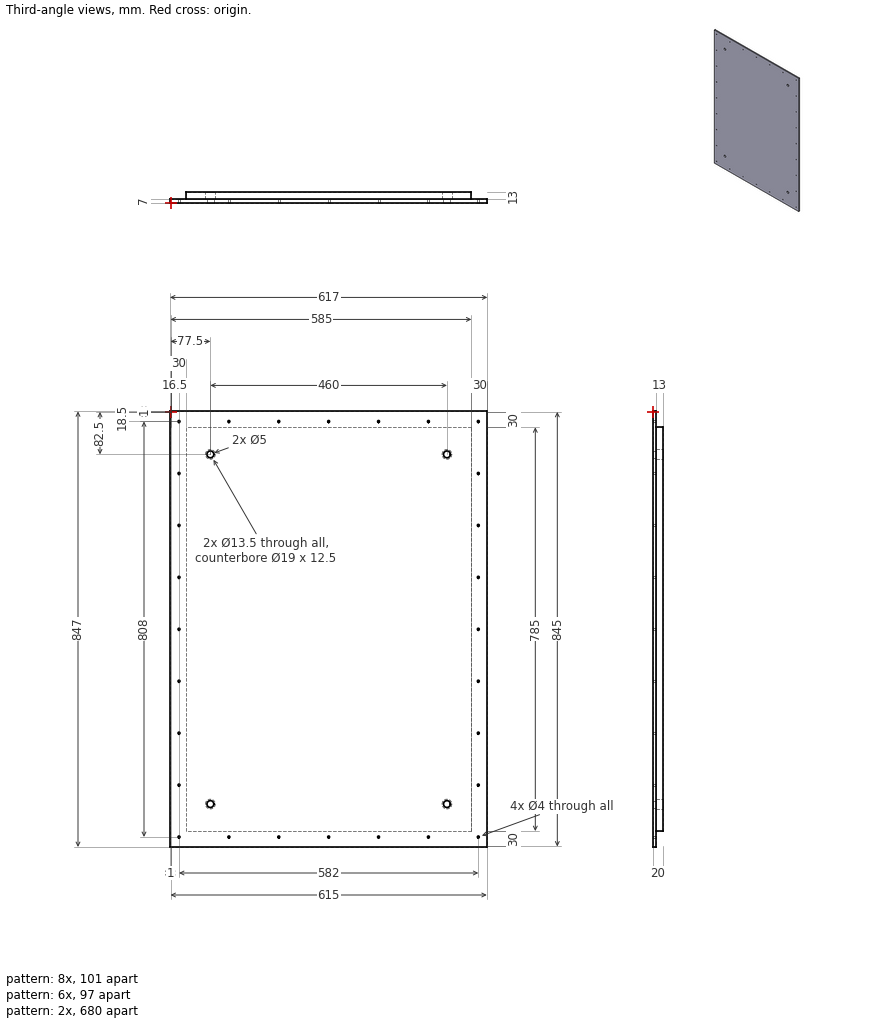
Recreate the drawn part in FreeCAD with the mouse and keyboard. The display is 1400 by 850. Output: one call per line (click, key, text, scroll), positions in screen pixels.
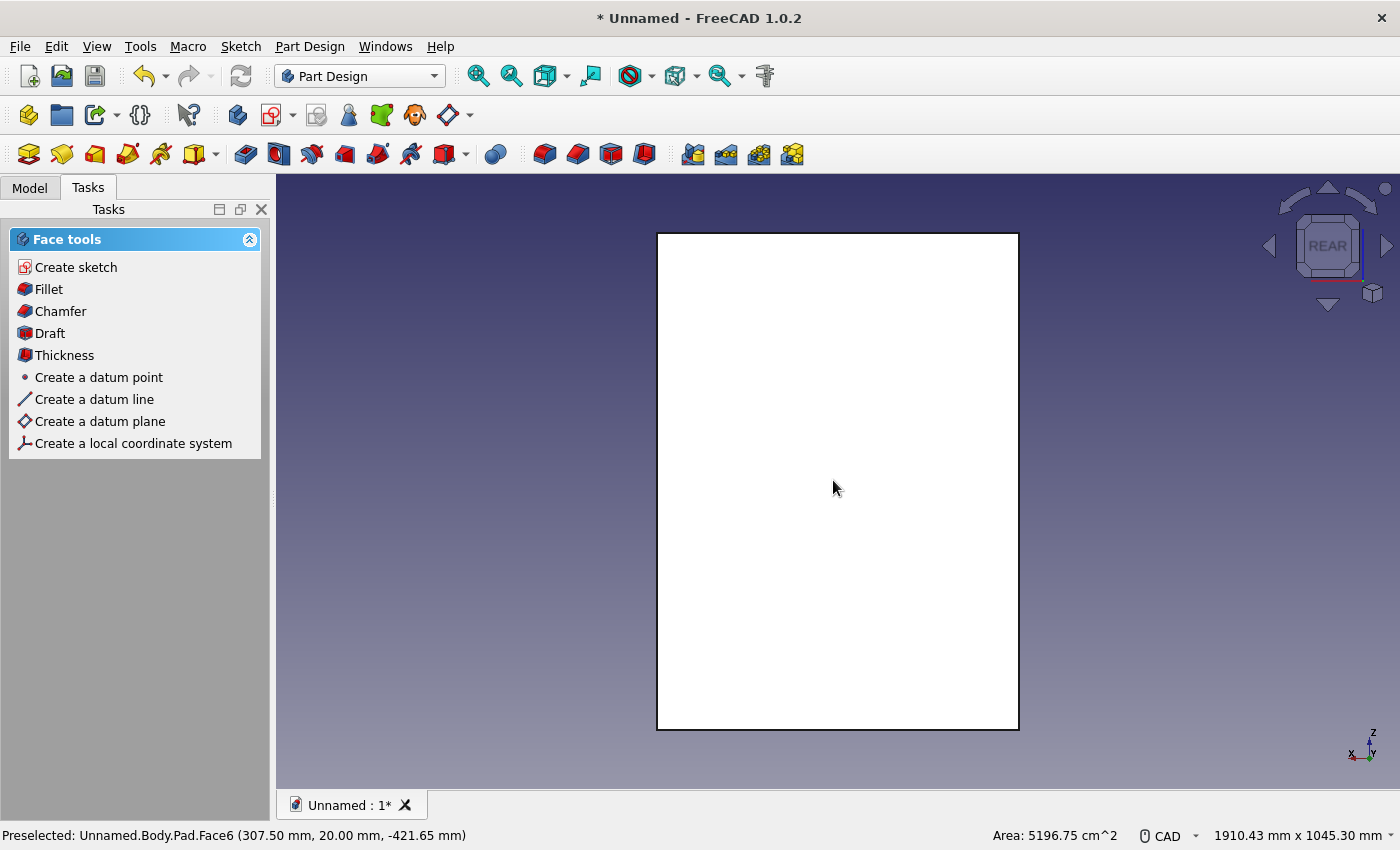
click(270, 116)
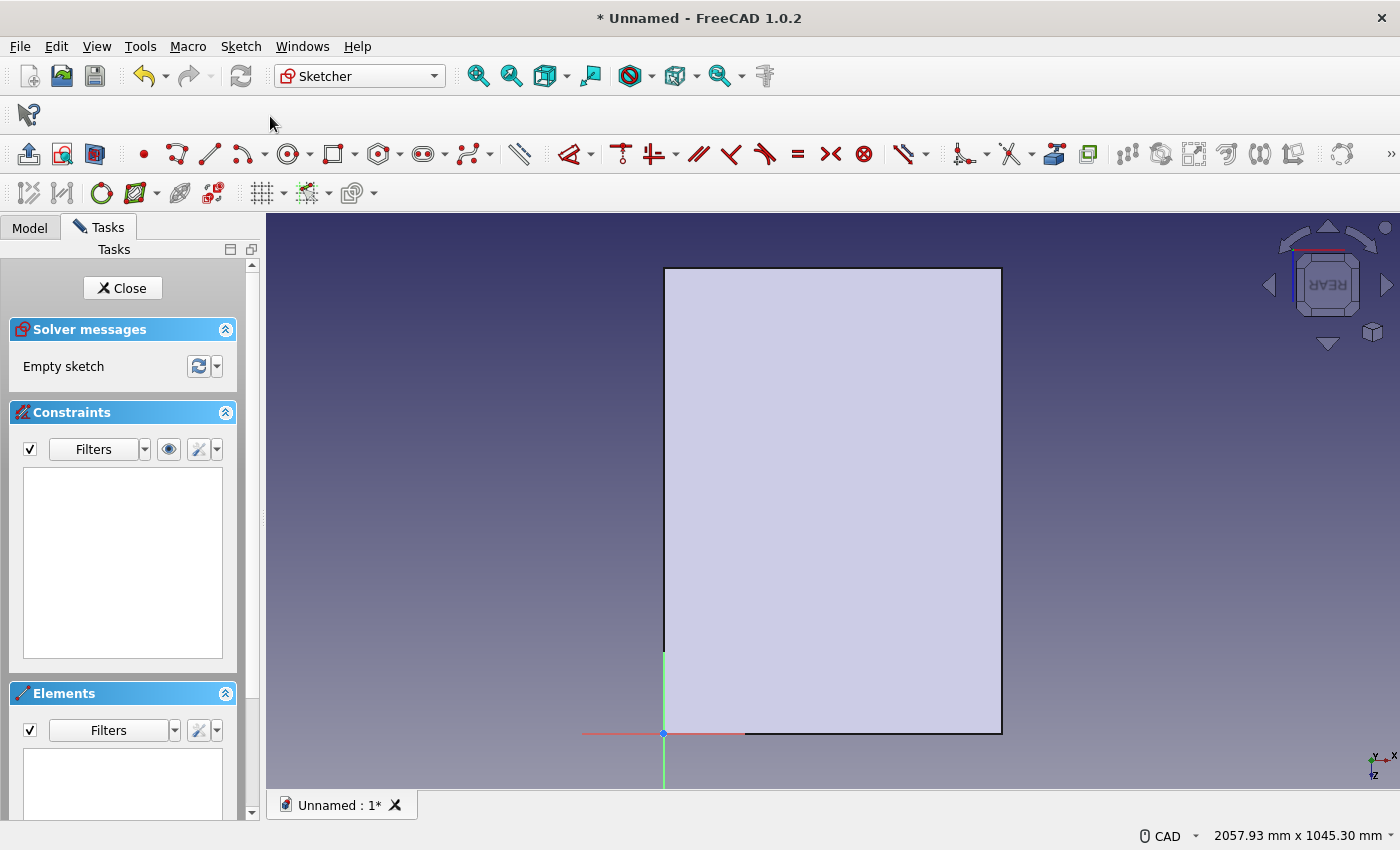
click(332, 154)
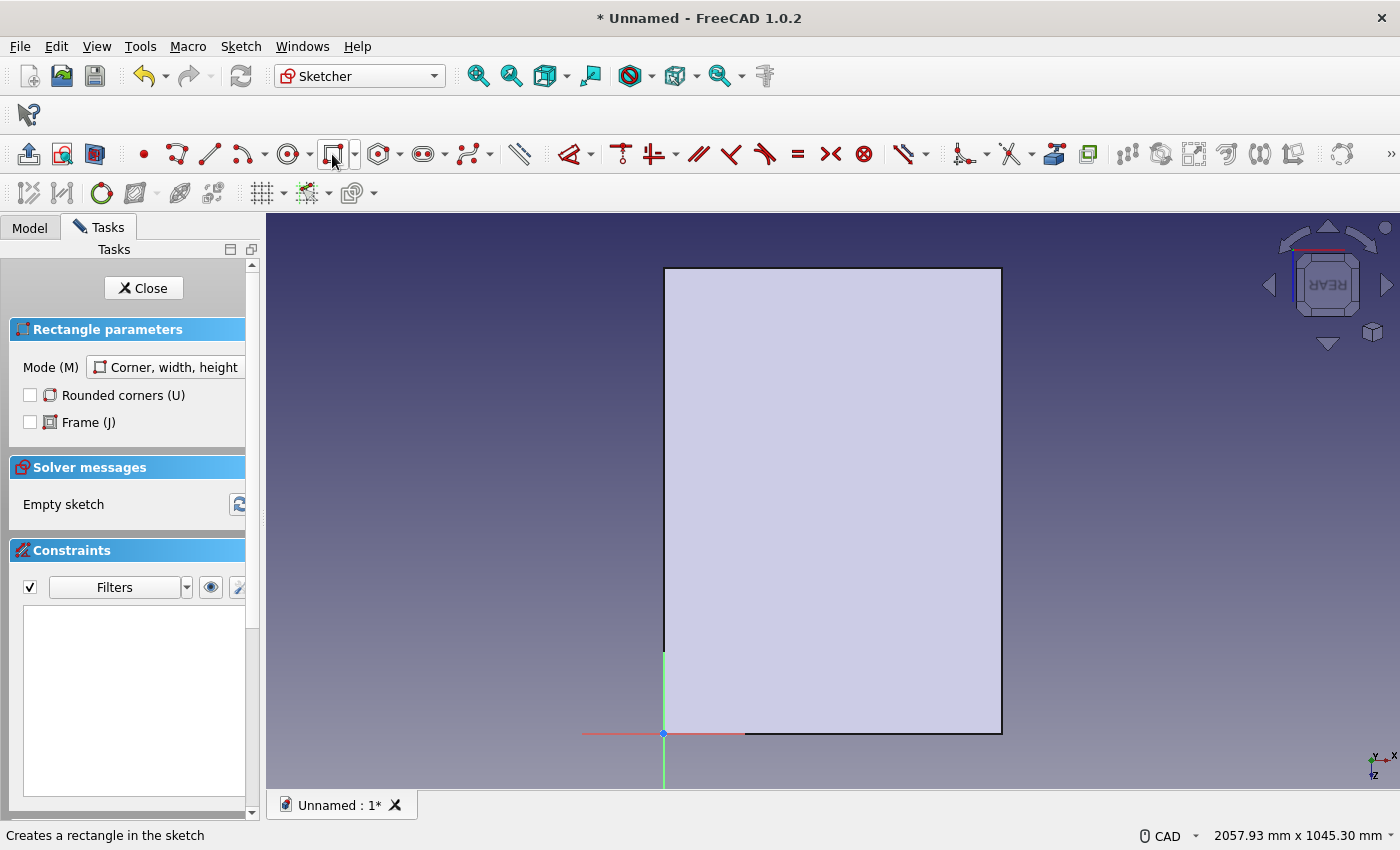
click(664, 268)
move(1002, 285)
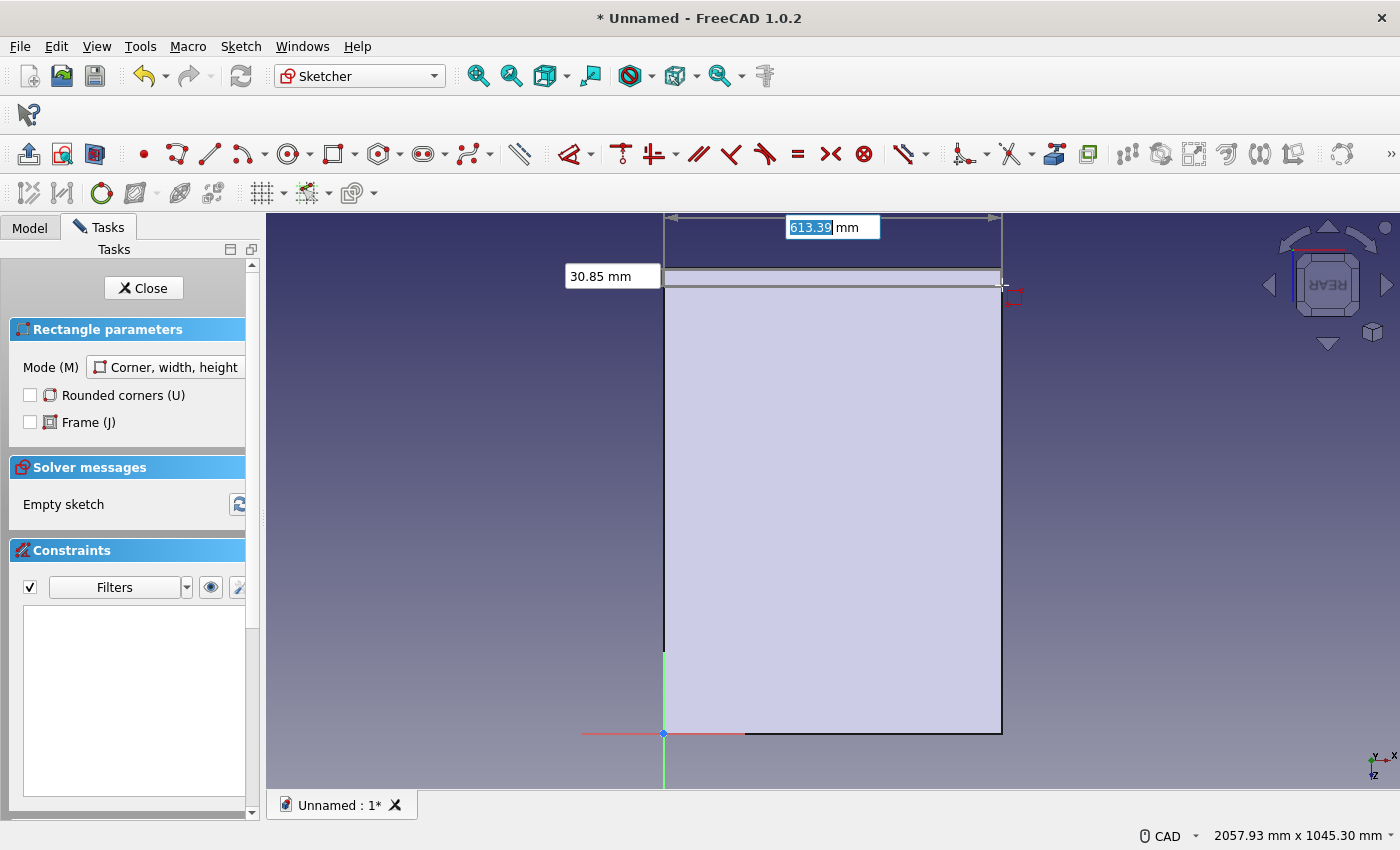
text(615)
key(Tab)
text(30)
key(Return)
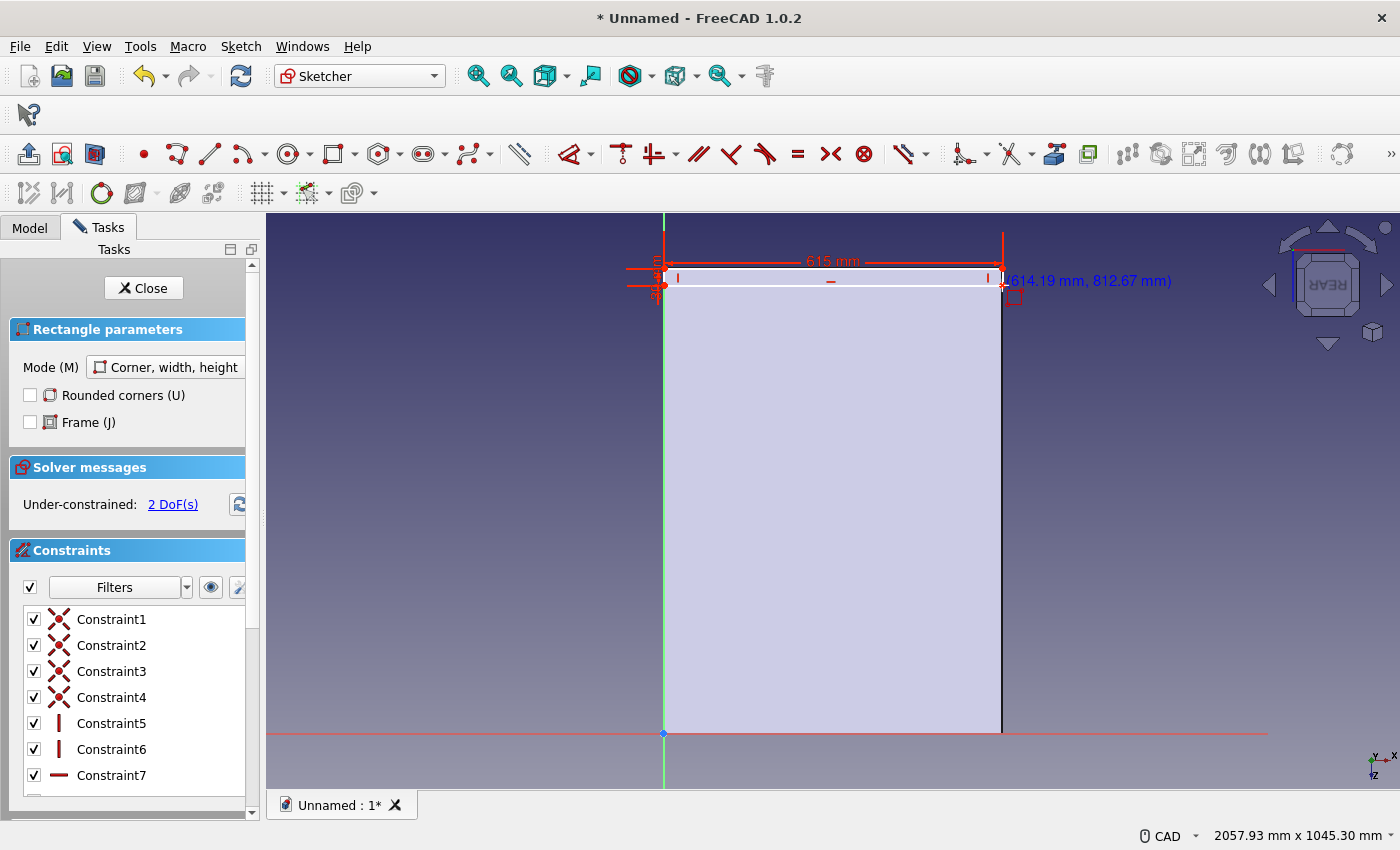
click(664, 734)
move(1002, 717)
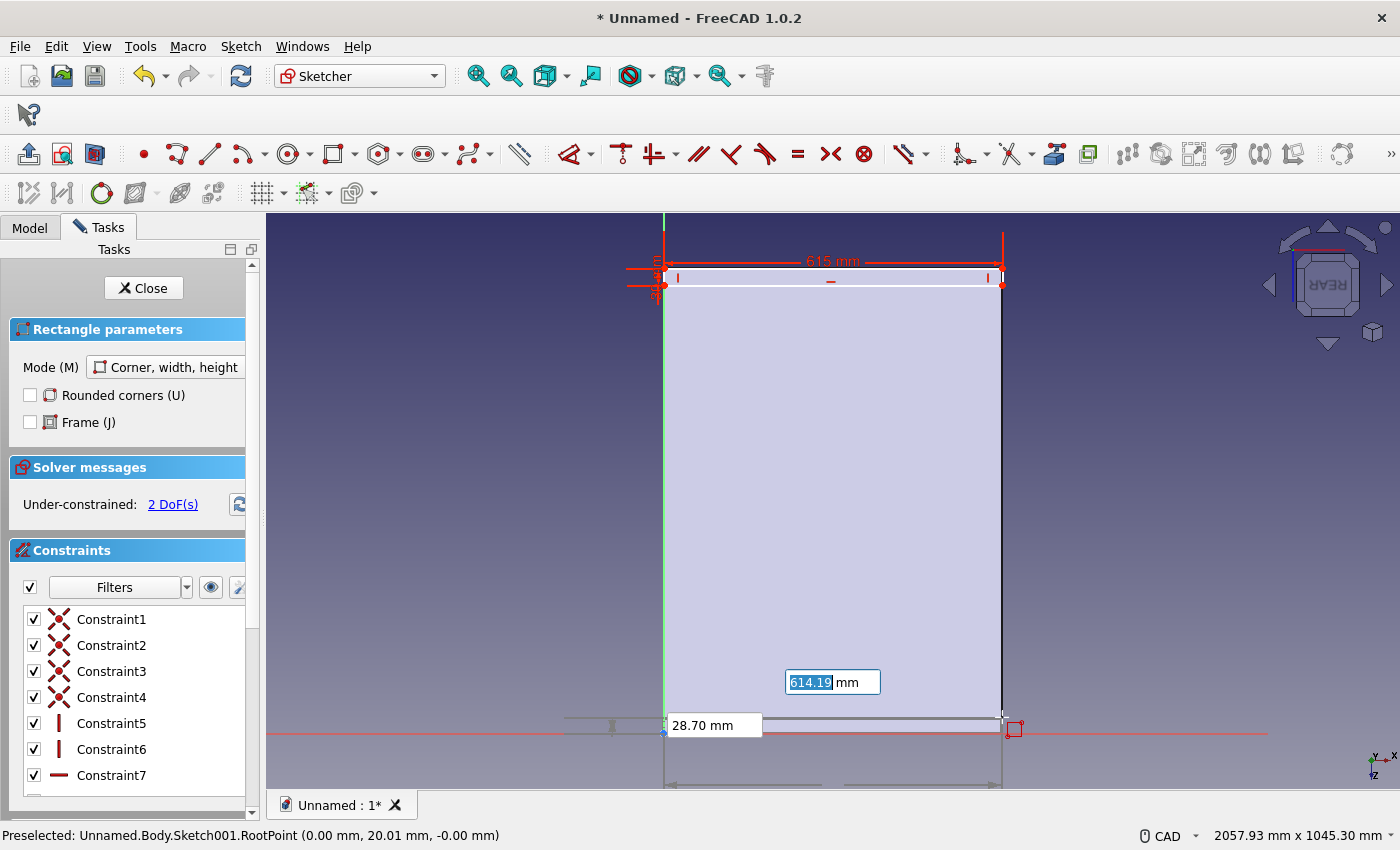
text(615)
key(Tab)
text(30)
key(Return)
key(Escape)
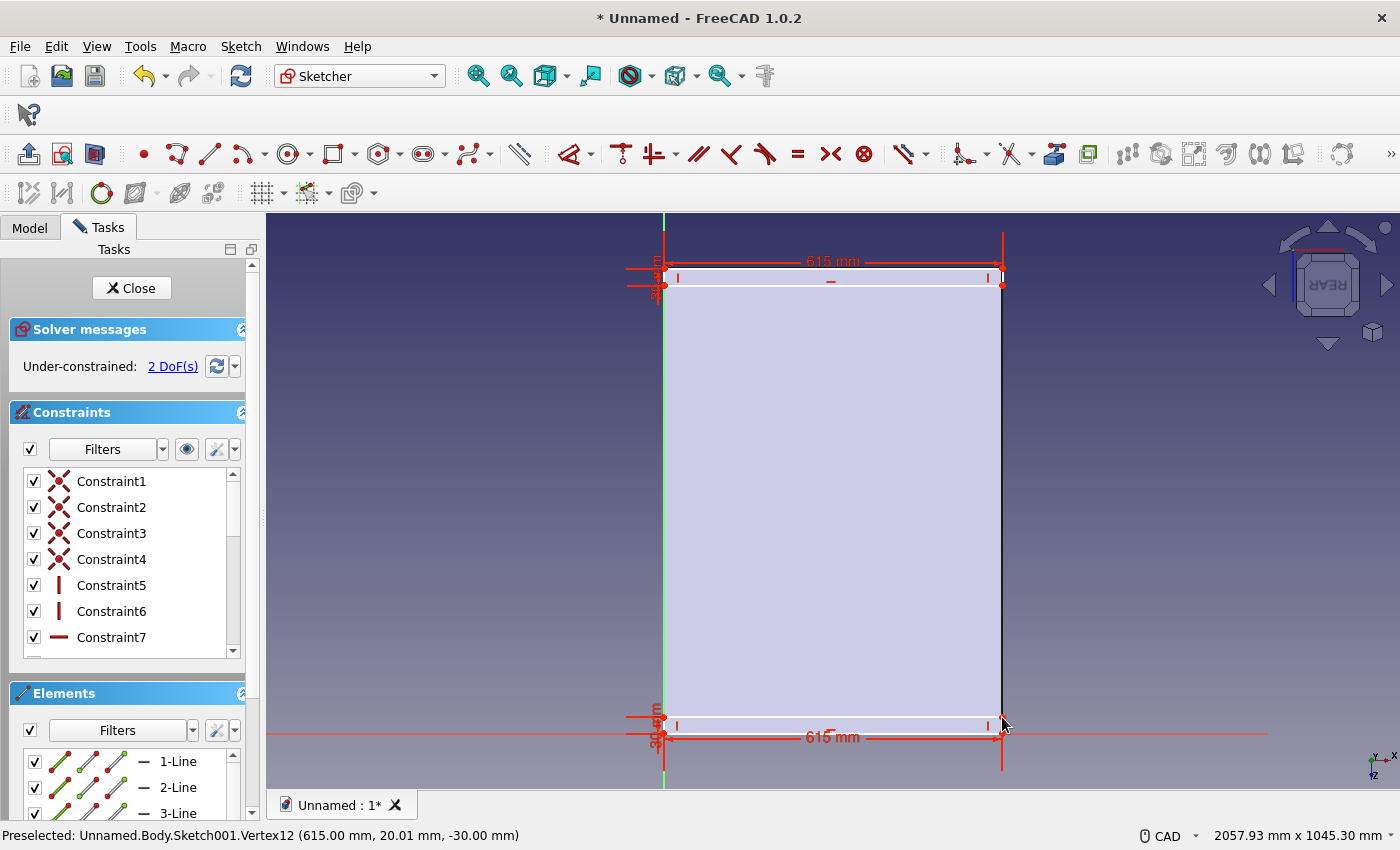
click(664, 269)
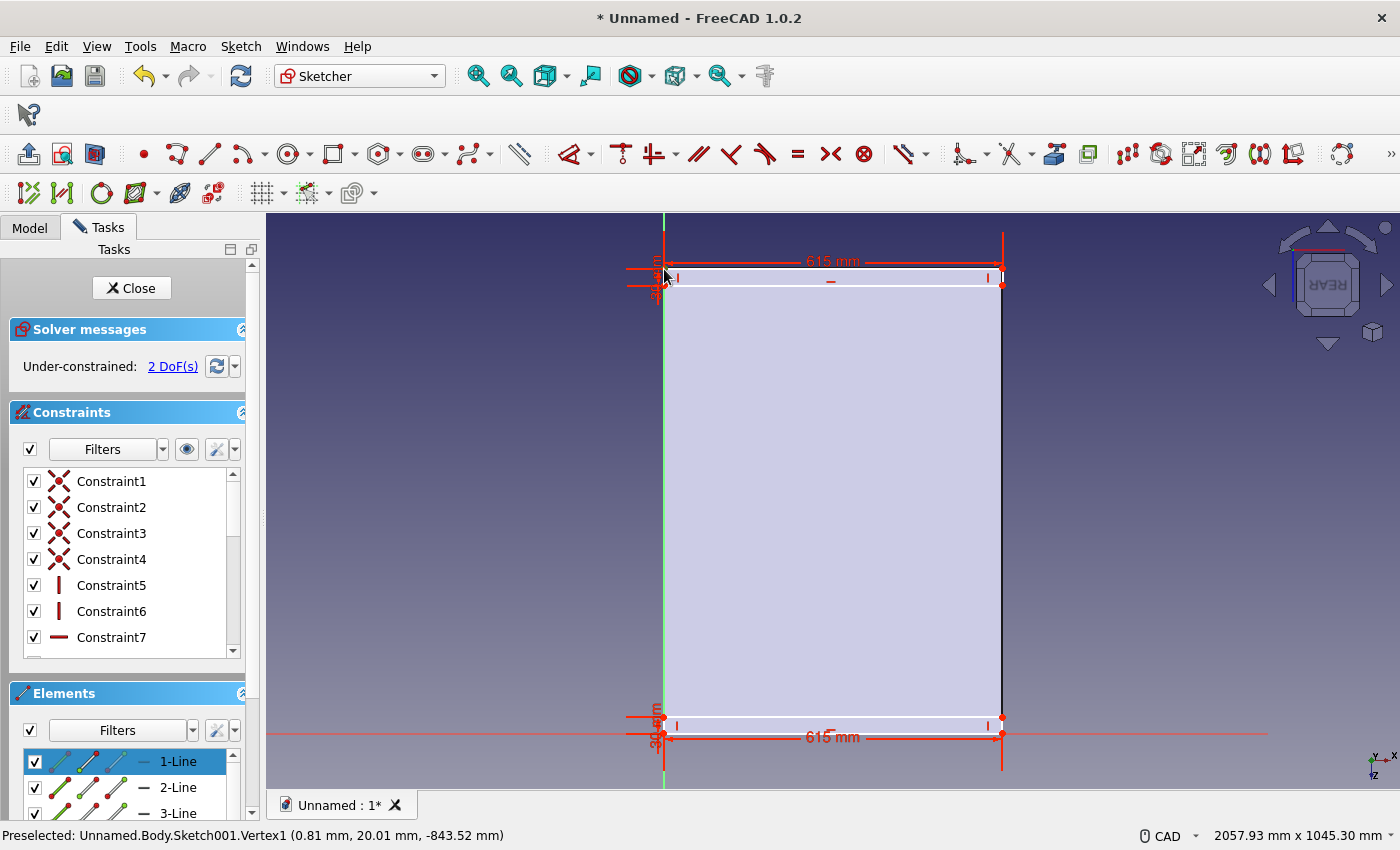
click(664, 687)